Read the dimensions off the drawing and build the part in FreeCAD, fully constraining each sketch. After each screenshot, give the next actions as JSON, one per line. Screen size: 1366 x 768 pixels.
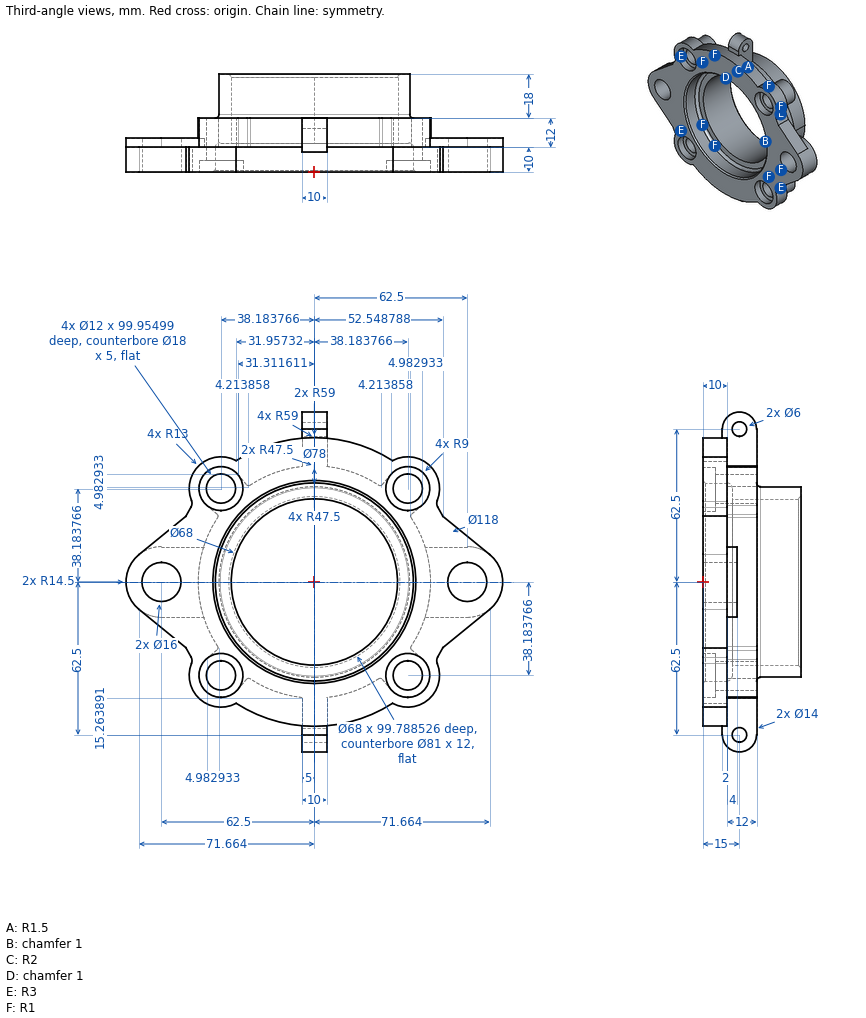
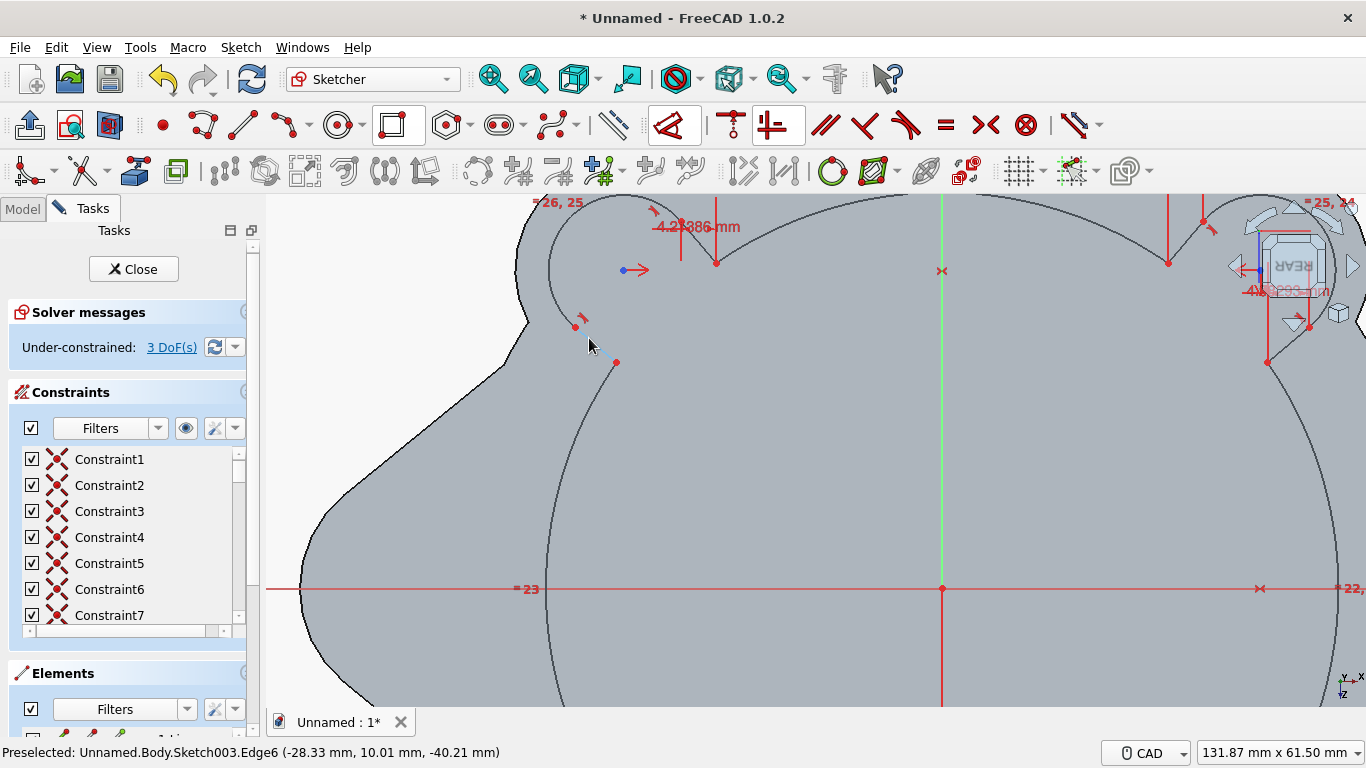
{"action": "left_click", "coordinate": [588, 338]}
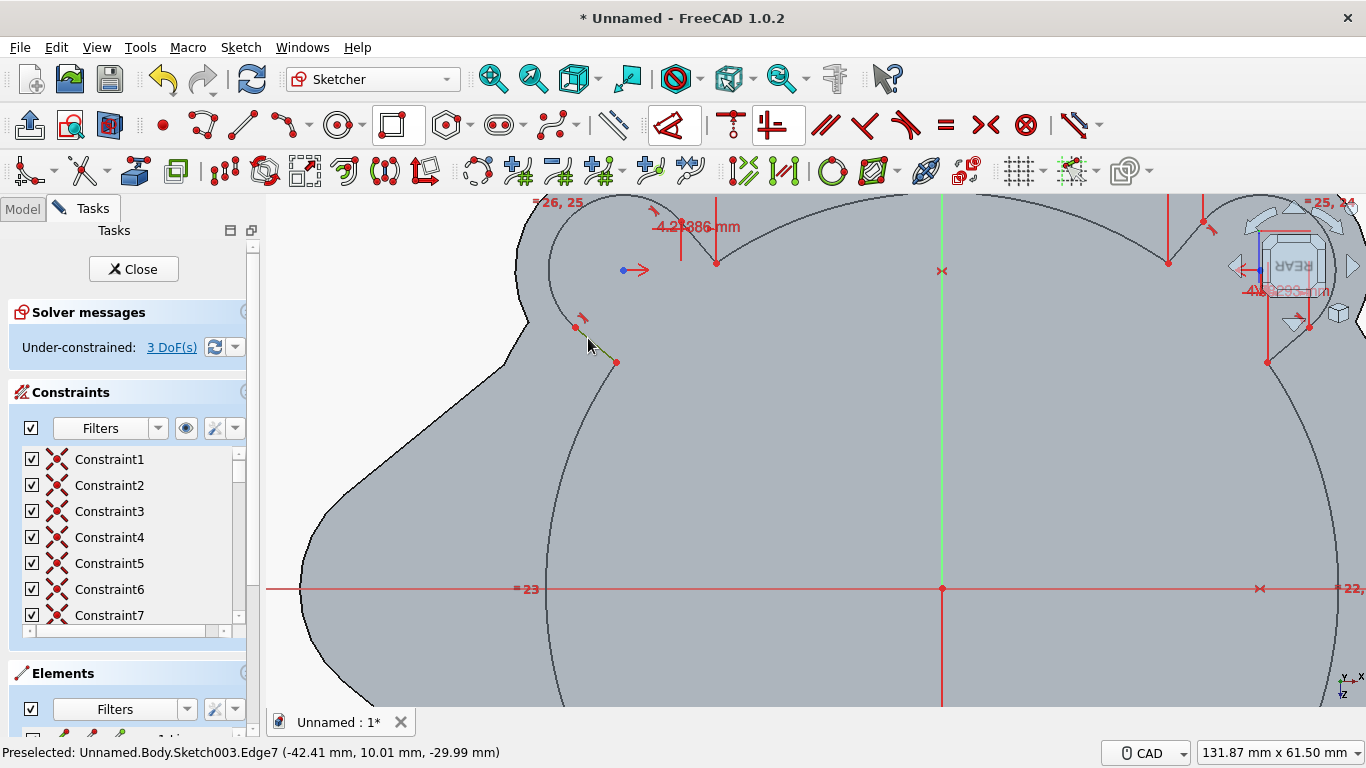
{"action": "left_click", "coordinate": [696, 126]}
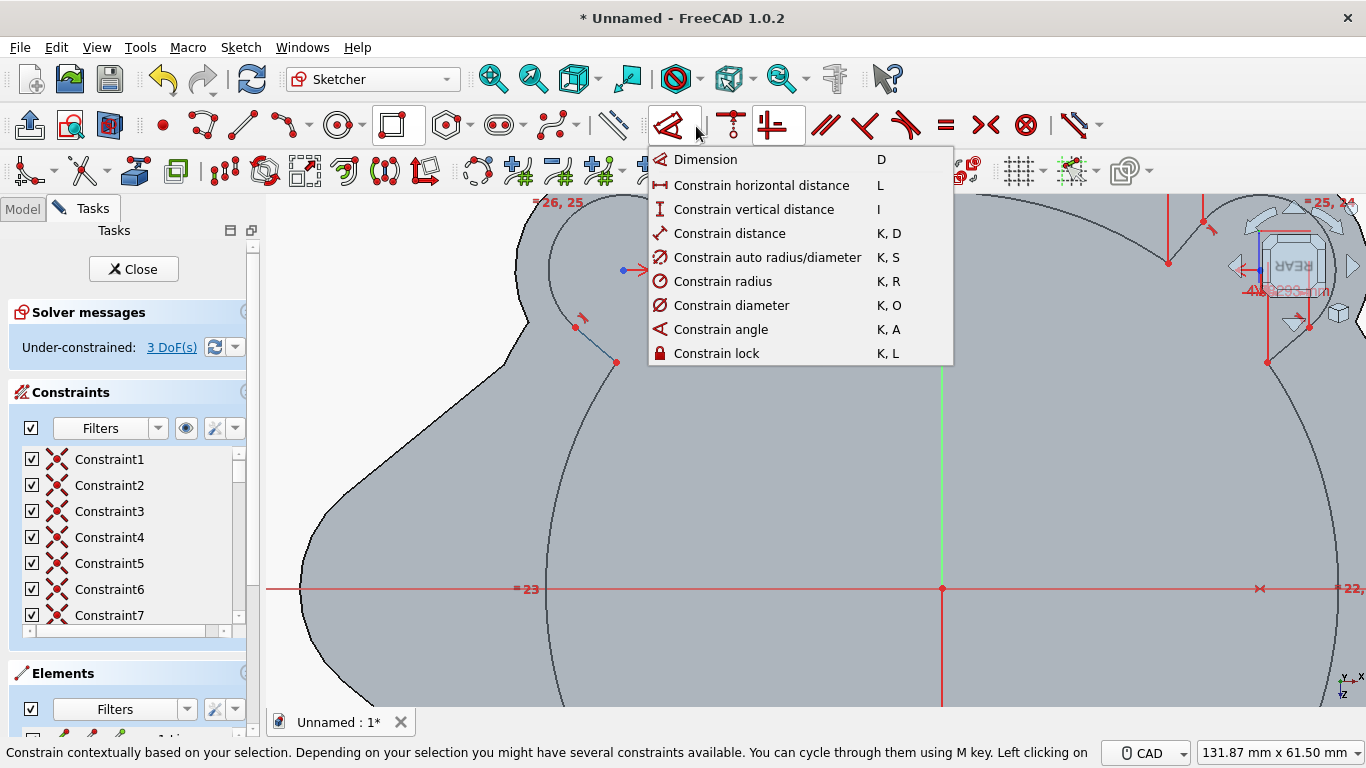
{"action": "left_click", "coordinate": [801, 185]}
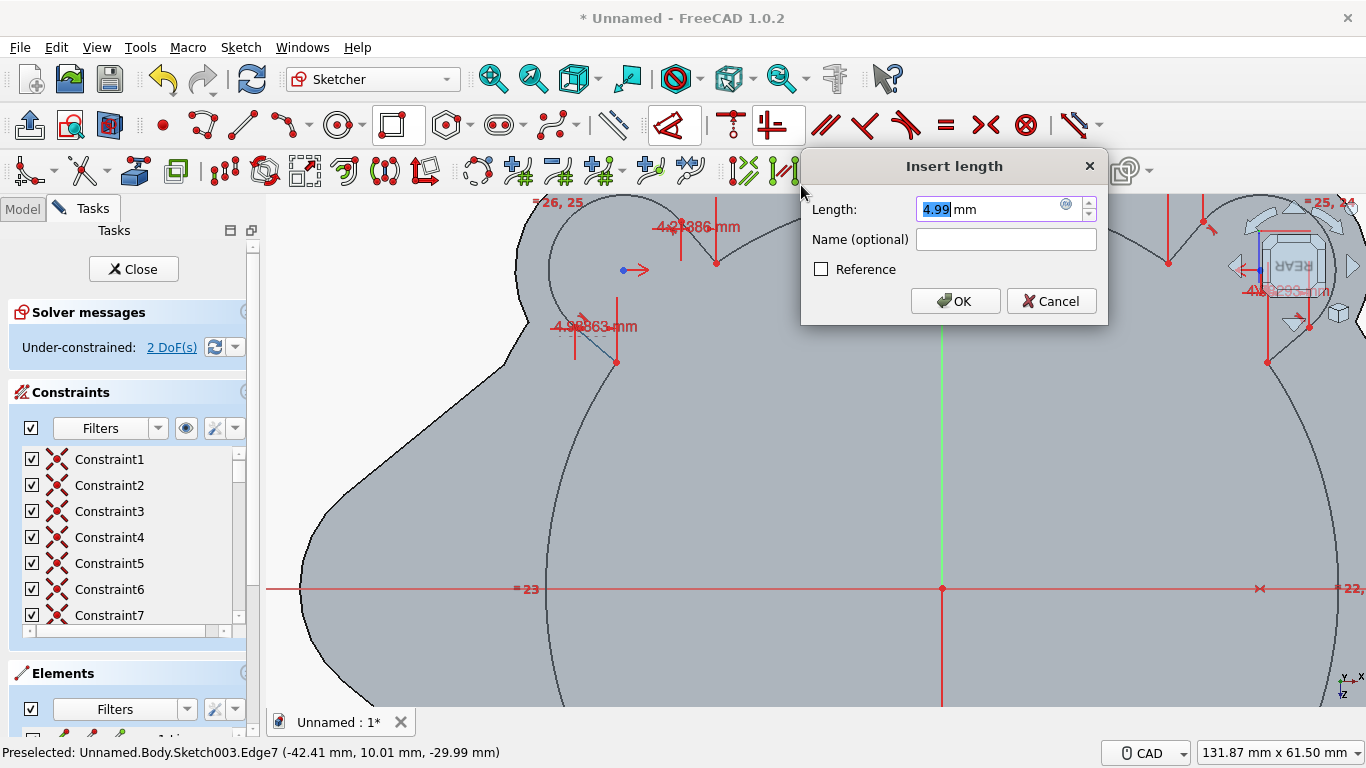
{"action": "type", "text": "4.982933"}
{"action": "key", "text": "Return"}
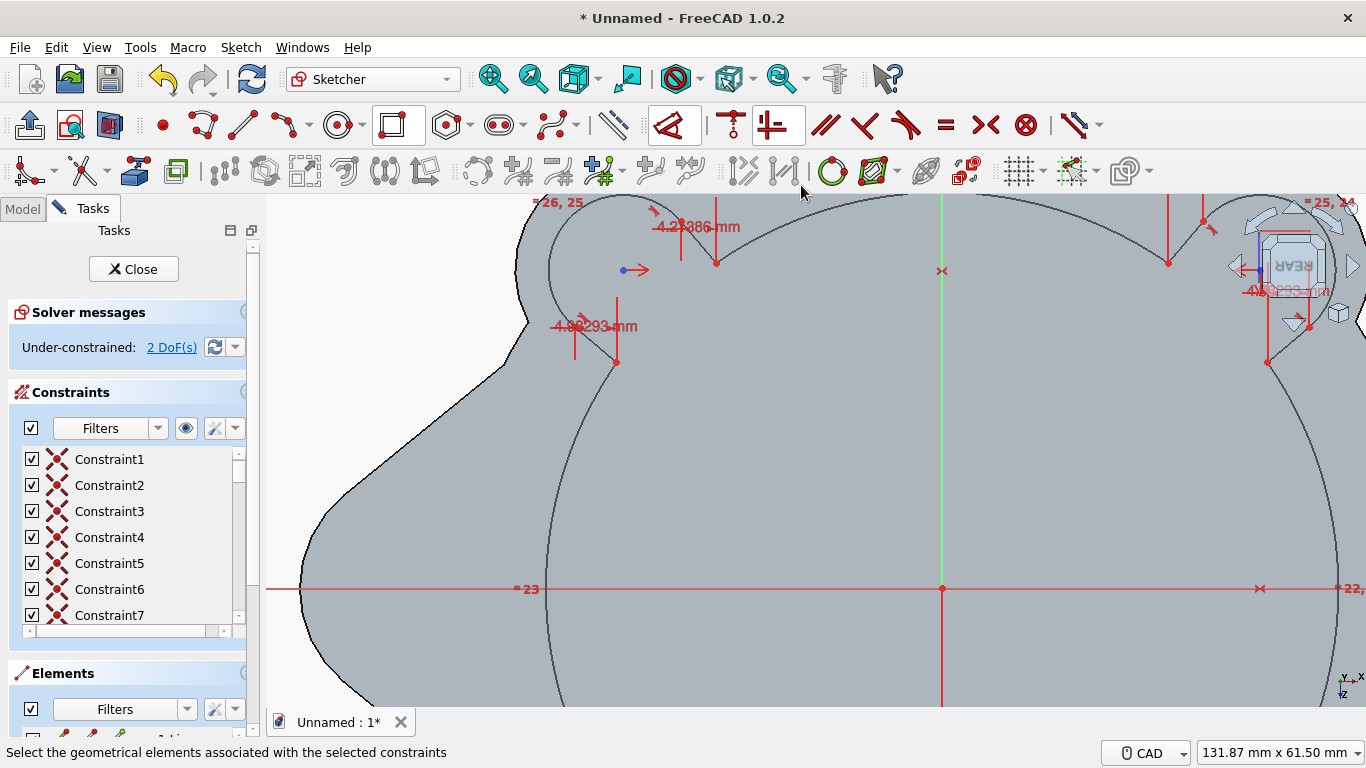
{"action": "scroll", "coordinate": [589, 338], "scroll_direction": "down", "scroll_amount": 4}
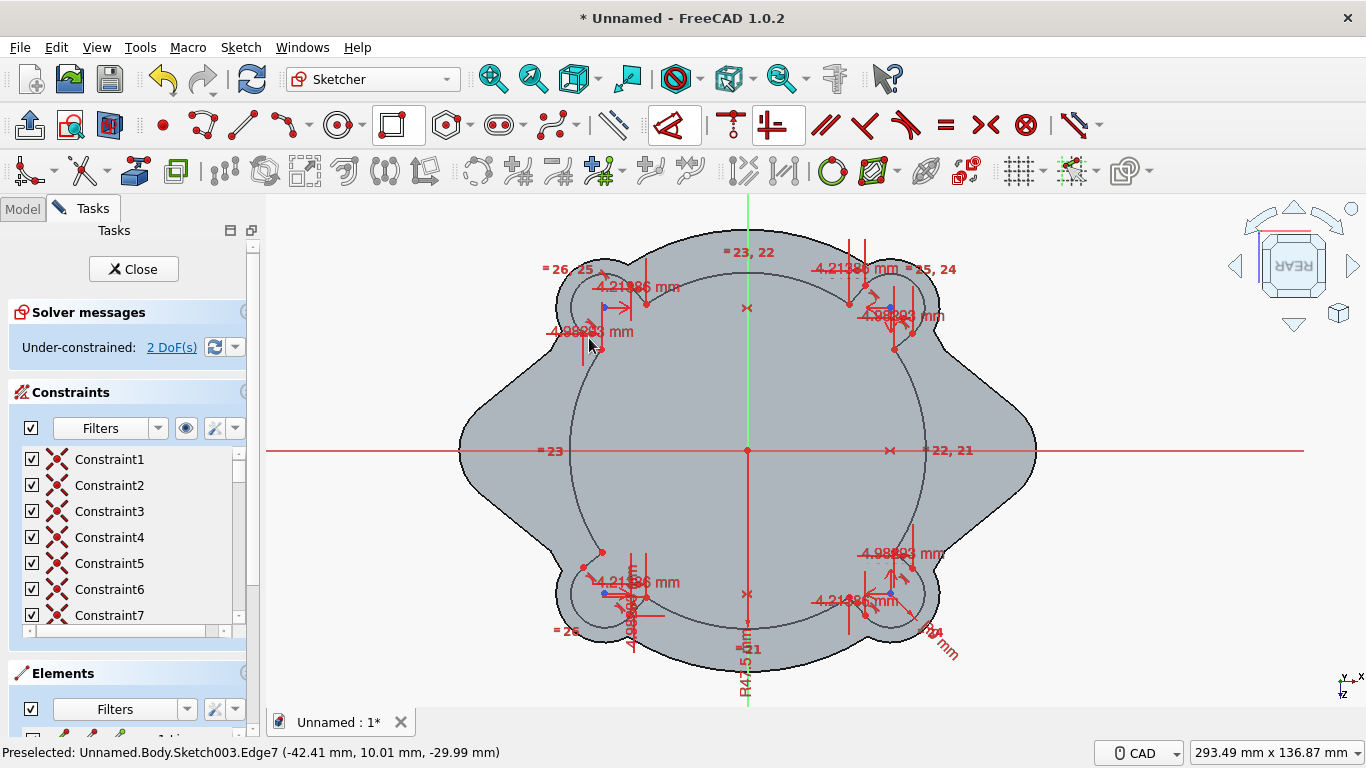
{"action": "scroll", "coordinate": [597, 557], "scroll_direction": "up", "scroll_amount": 4}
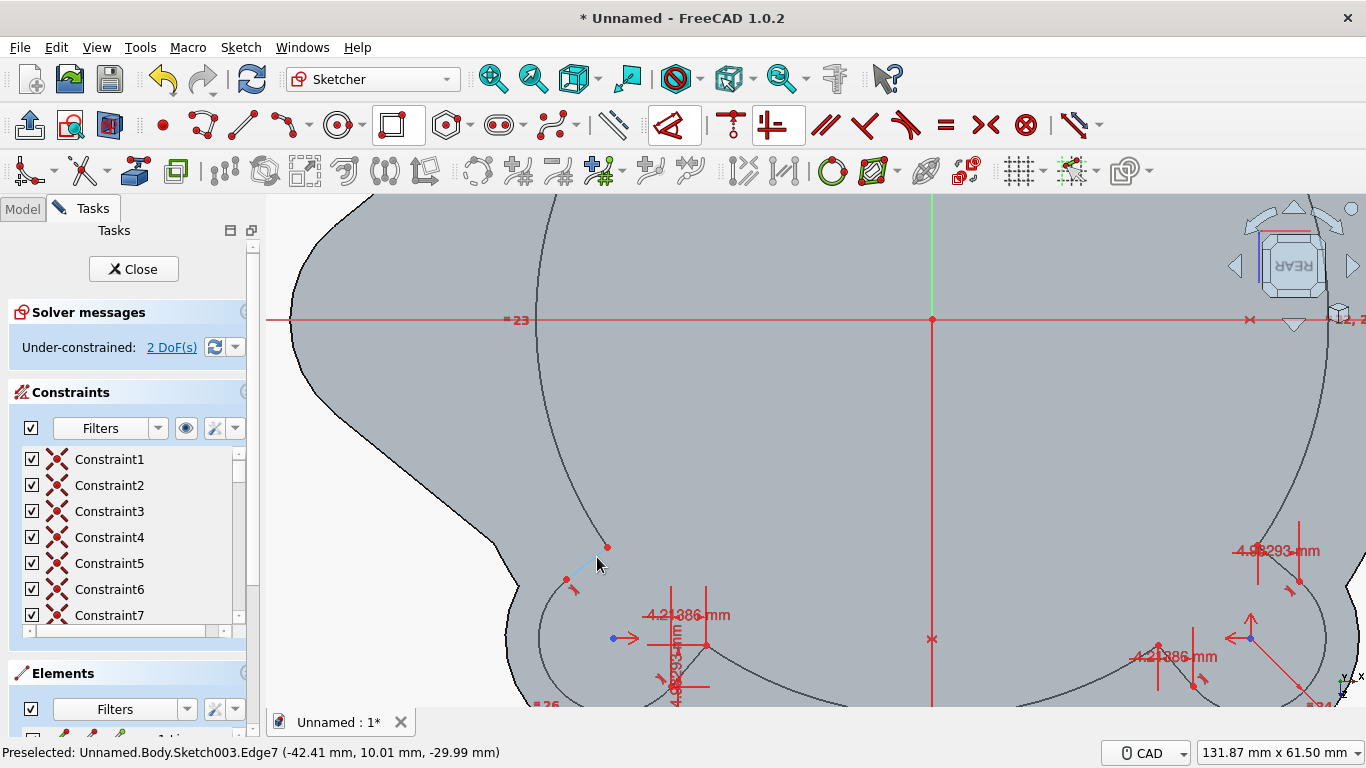
{"action": "left_click", "coordinate": [596, 557]}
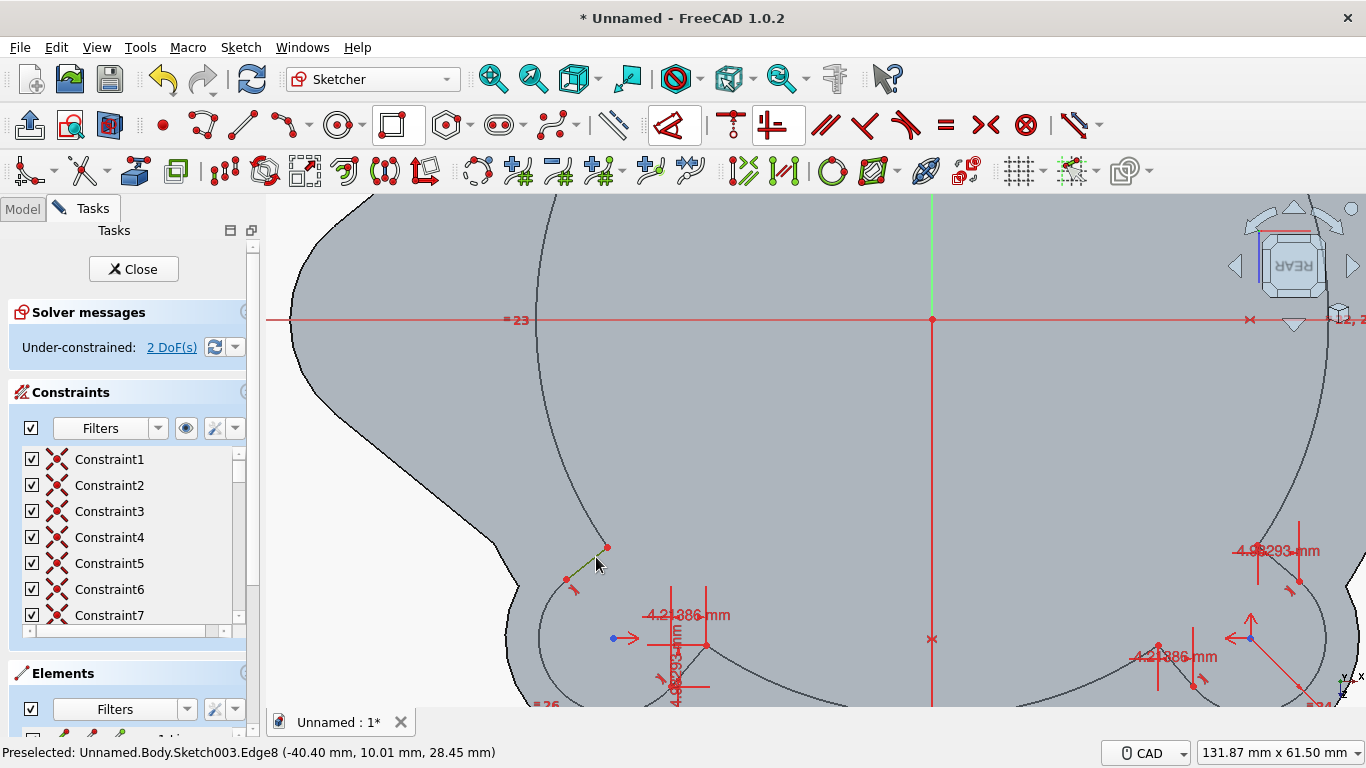
{"action": "key", "text": "l"}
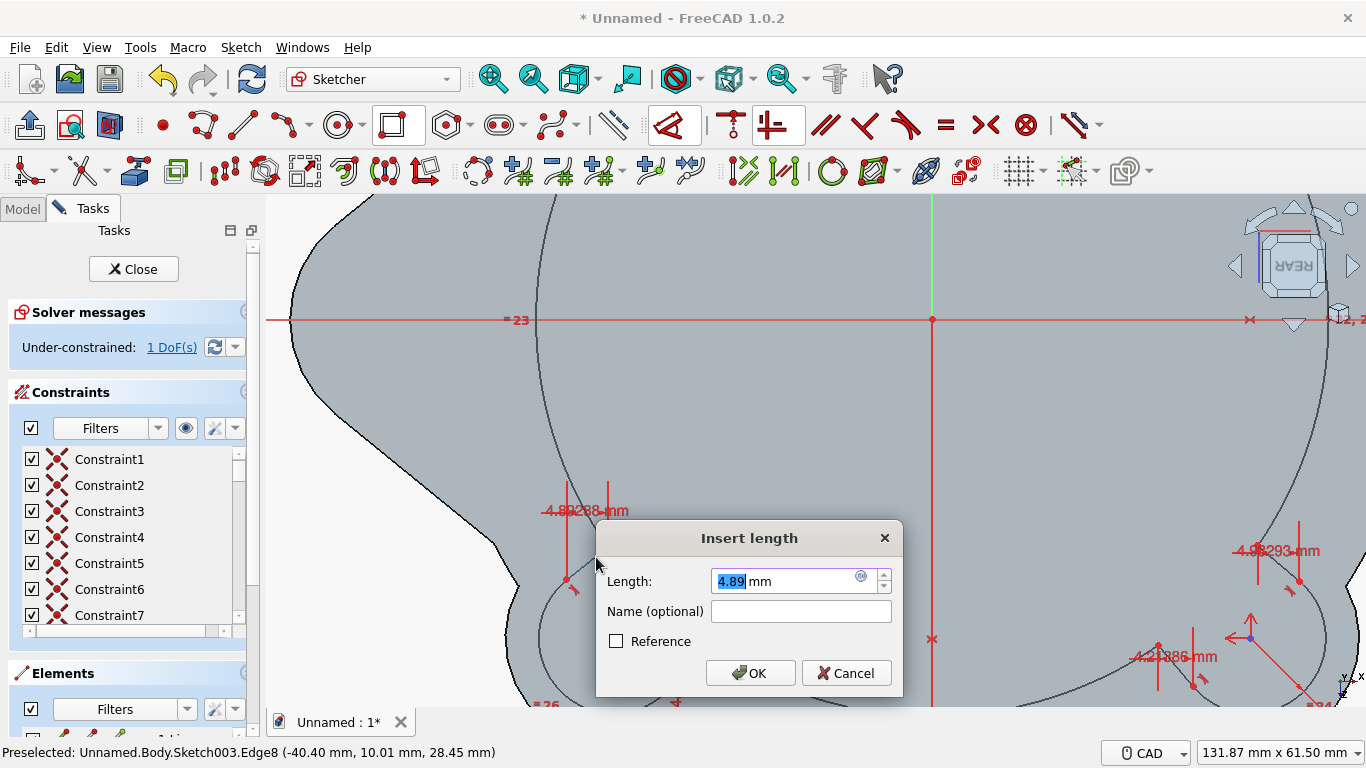
{"action": "type", "text": "4.982933"}
{"action": "key", "text": "Return"}